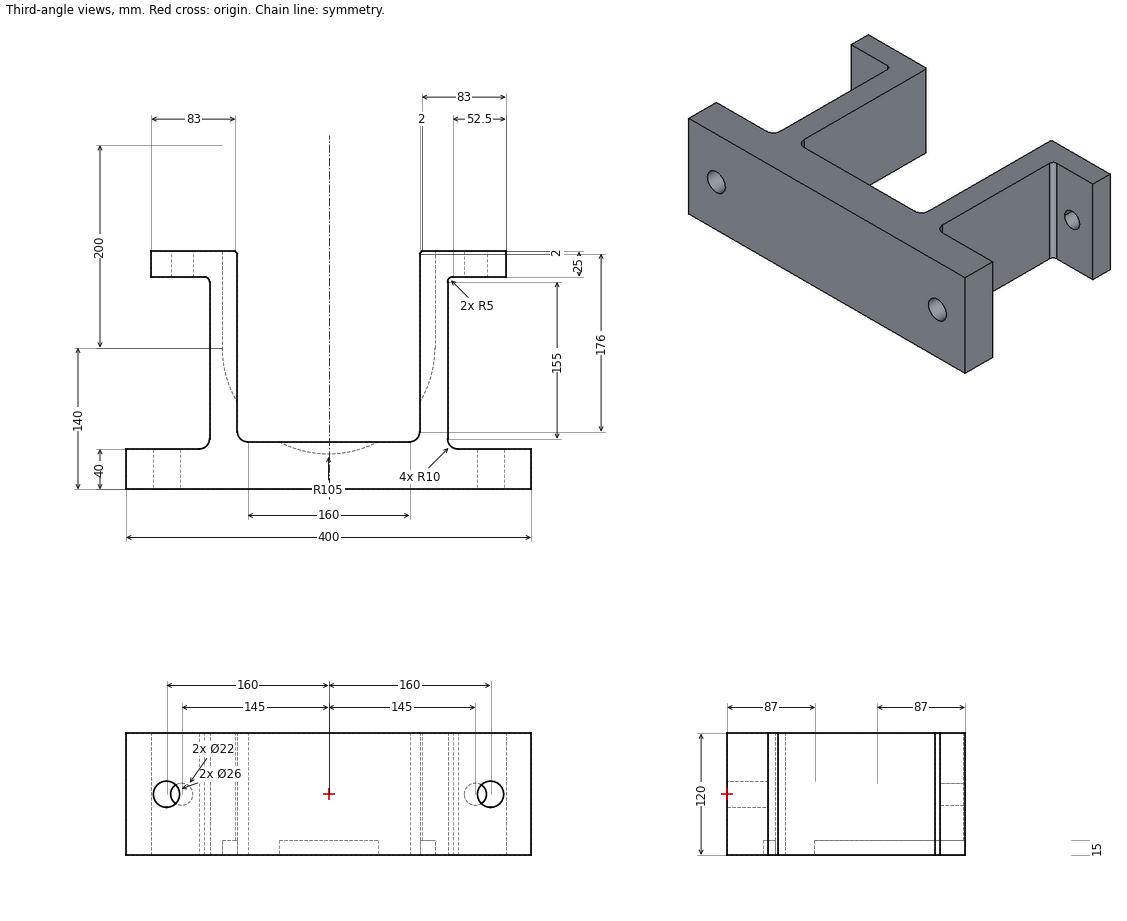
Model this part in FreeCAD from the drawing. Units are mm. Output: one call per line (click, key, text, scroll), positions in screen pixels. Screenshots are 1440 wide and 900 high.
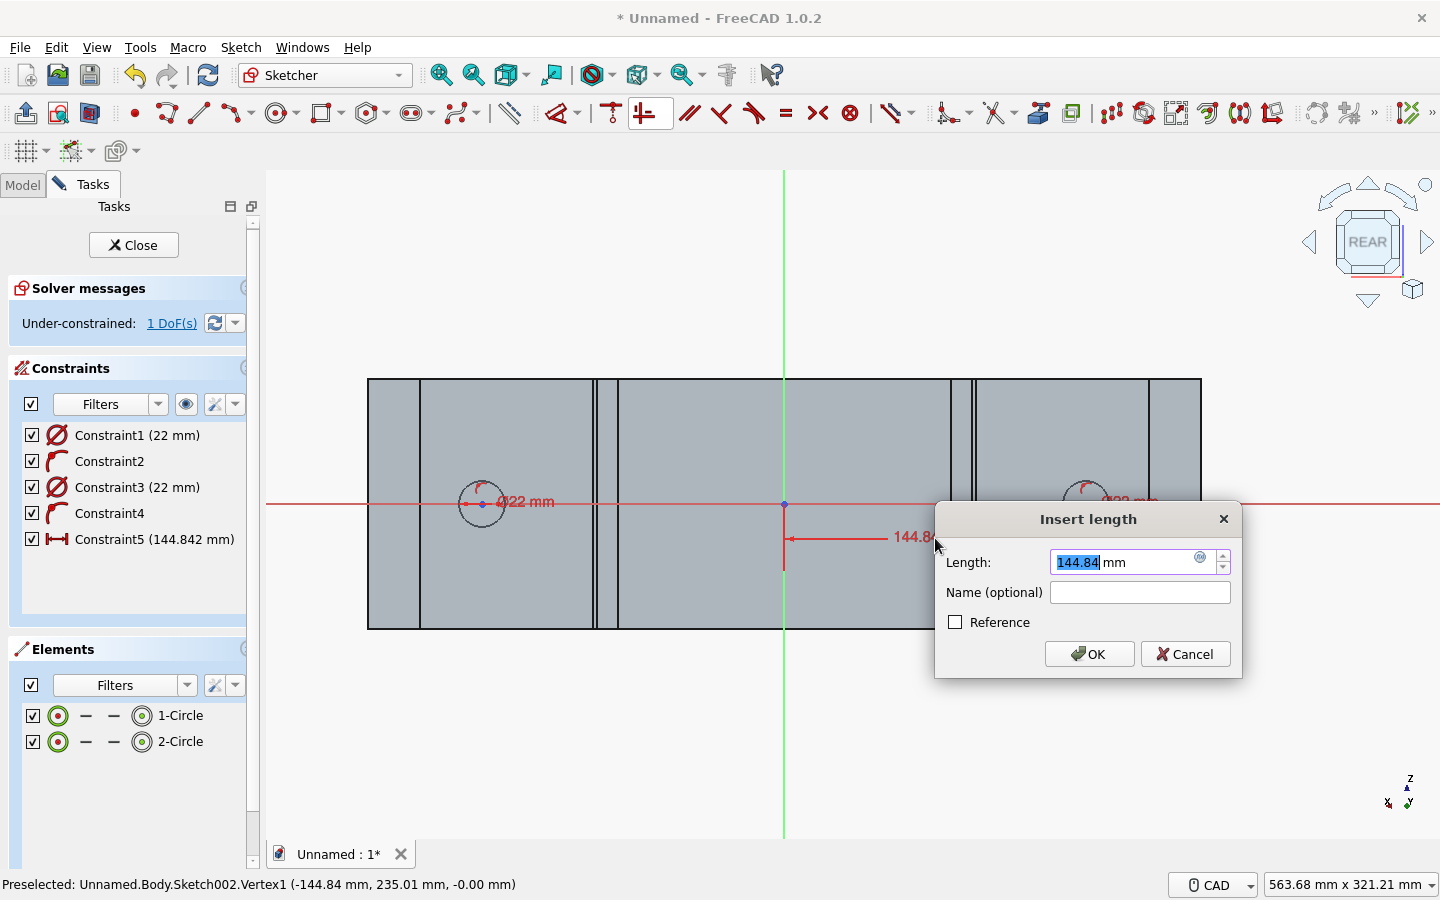
text(145)
key(Return)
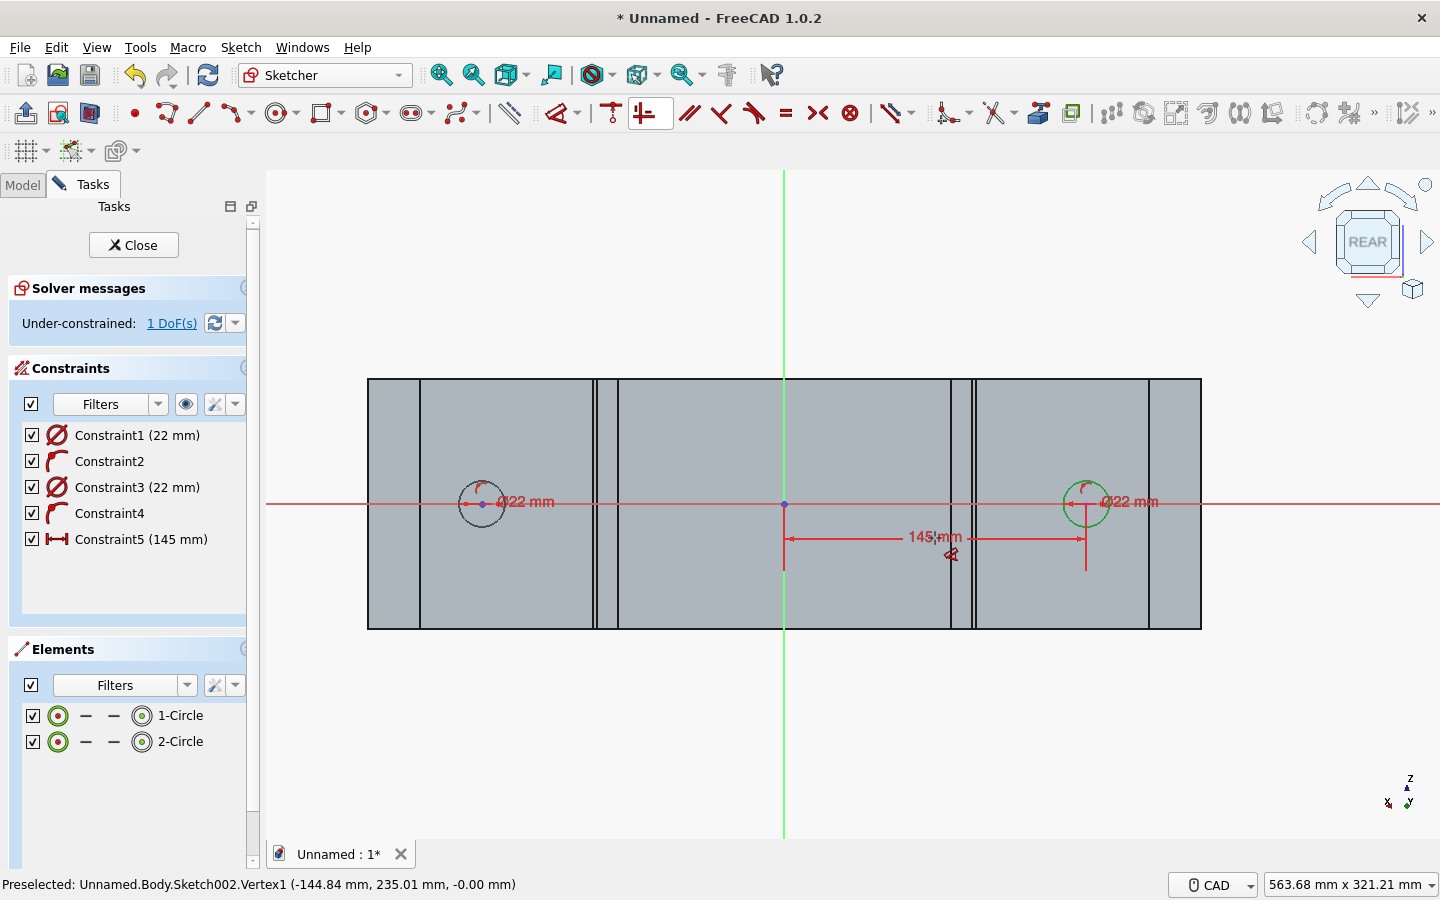
click(482, 504)
click(633, 538)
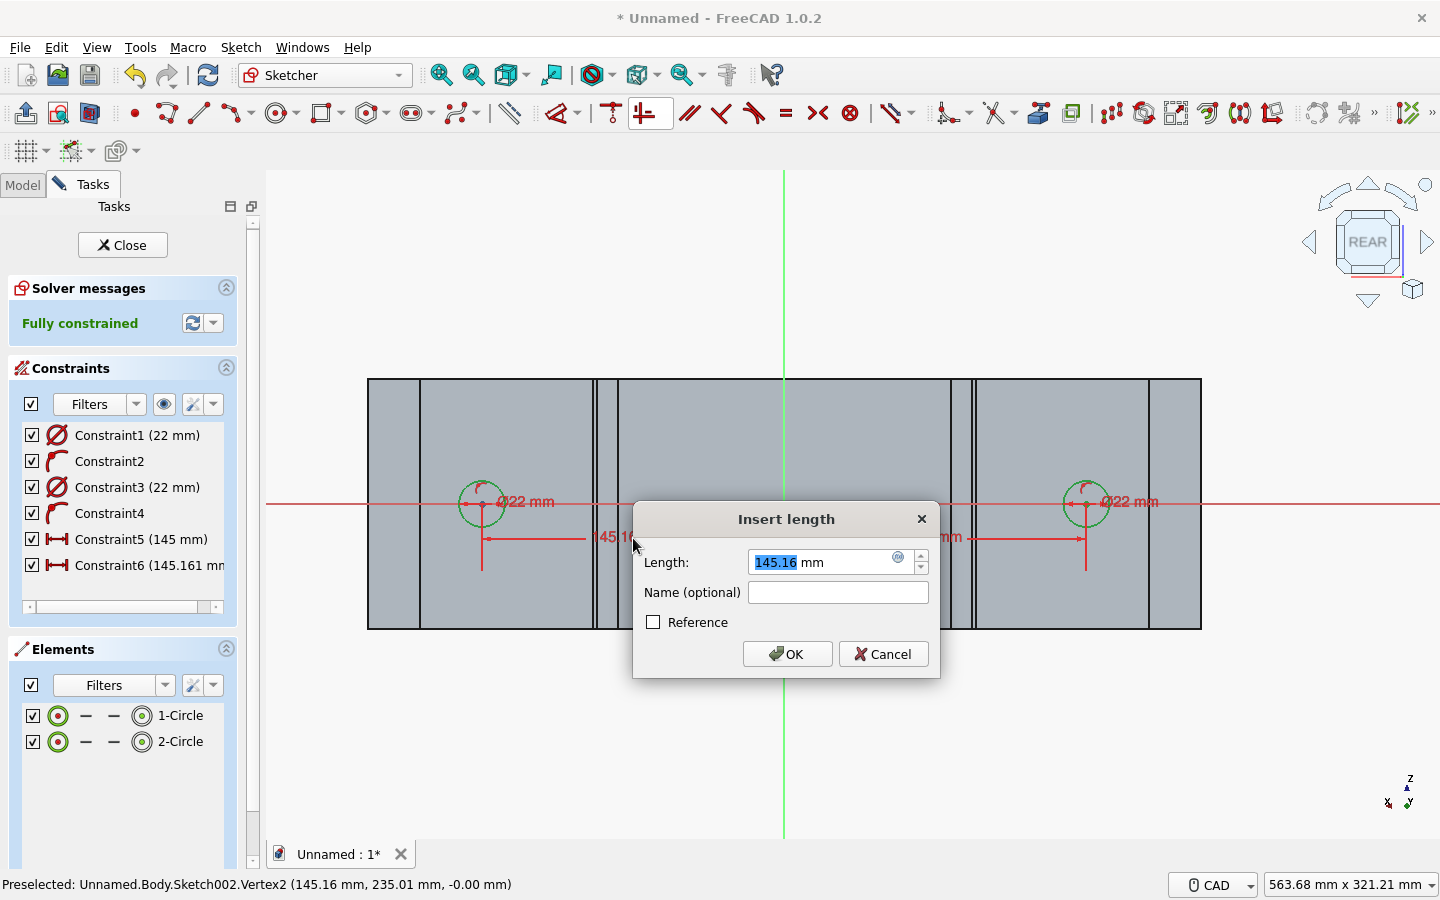
text(145)
key(Return)
key(Escape)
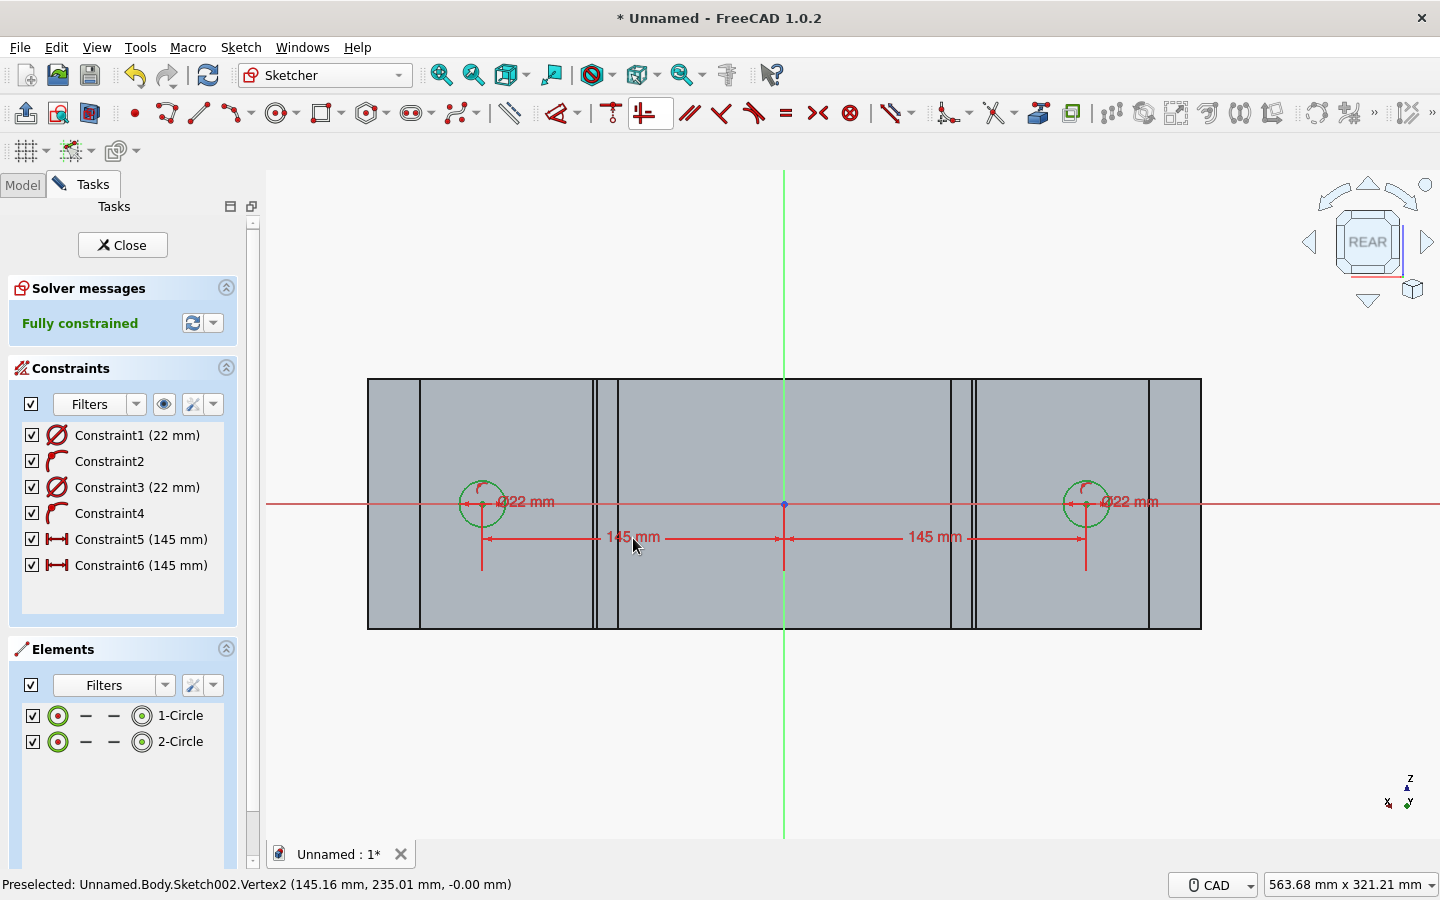
click(123, 245)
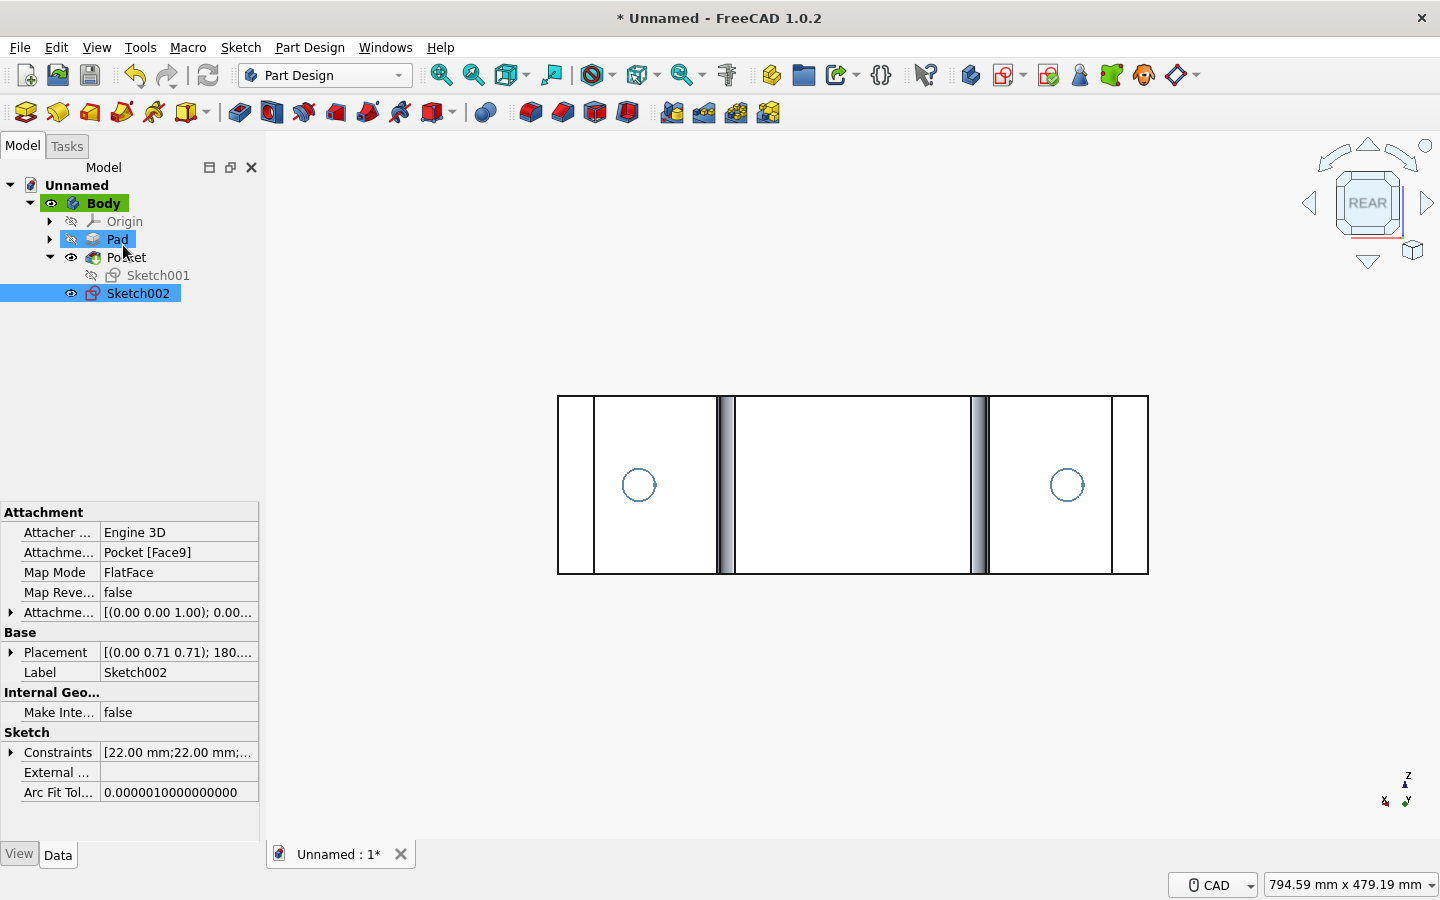
click(240, 112)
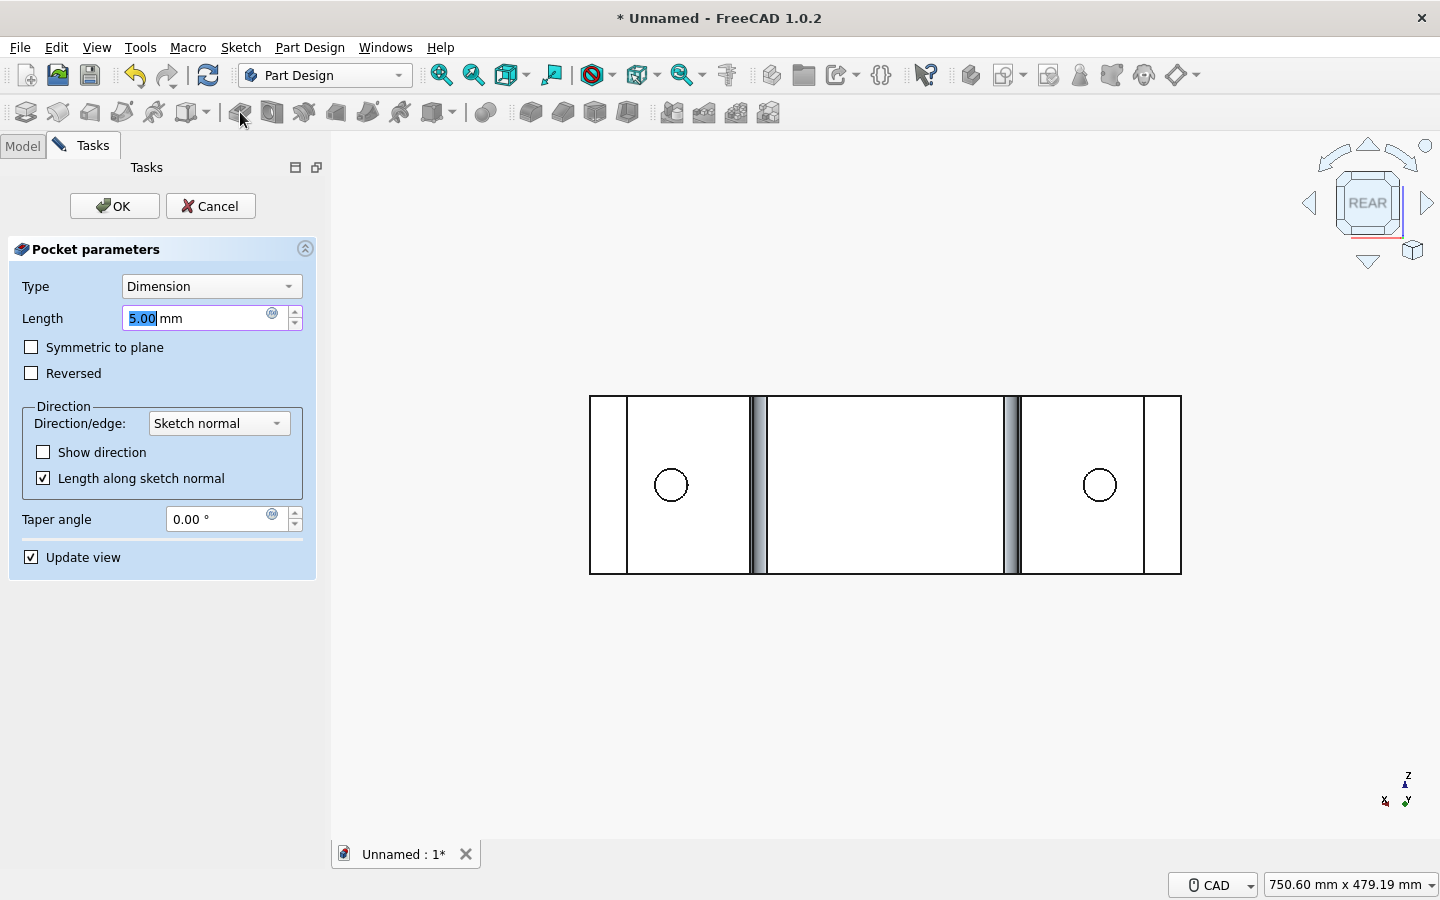
text(87)
key(Tab)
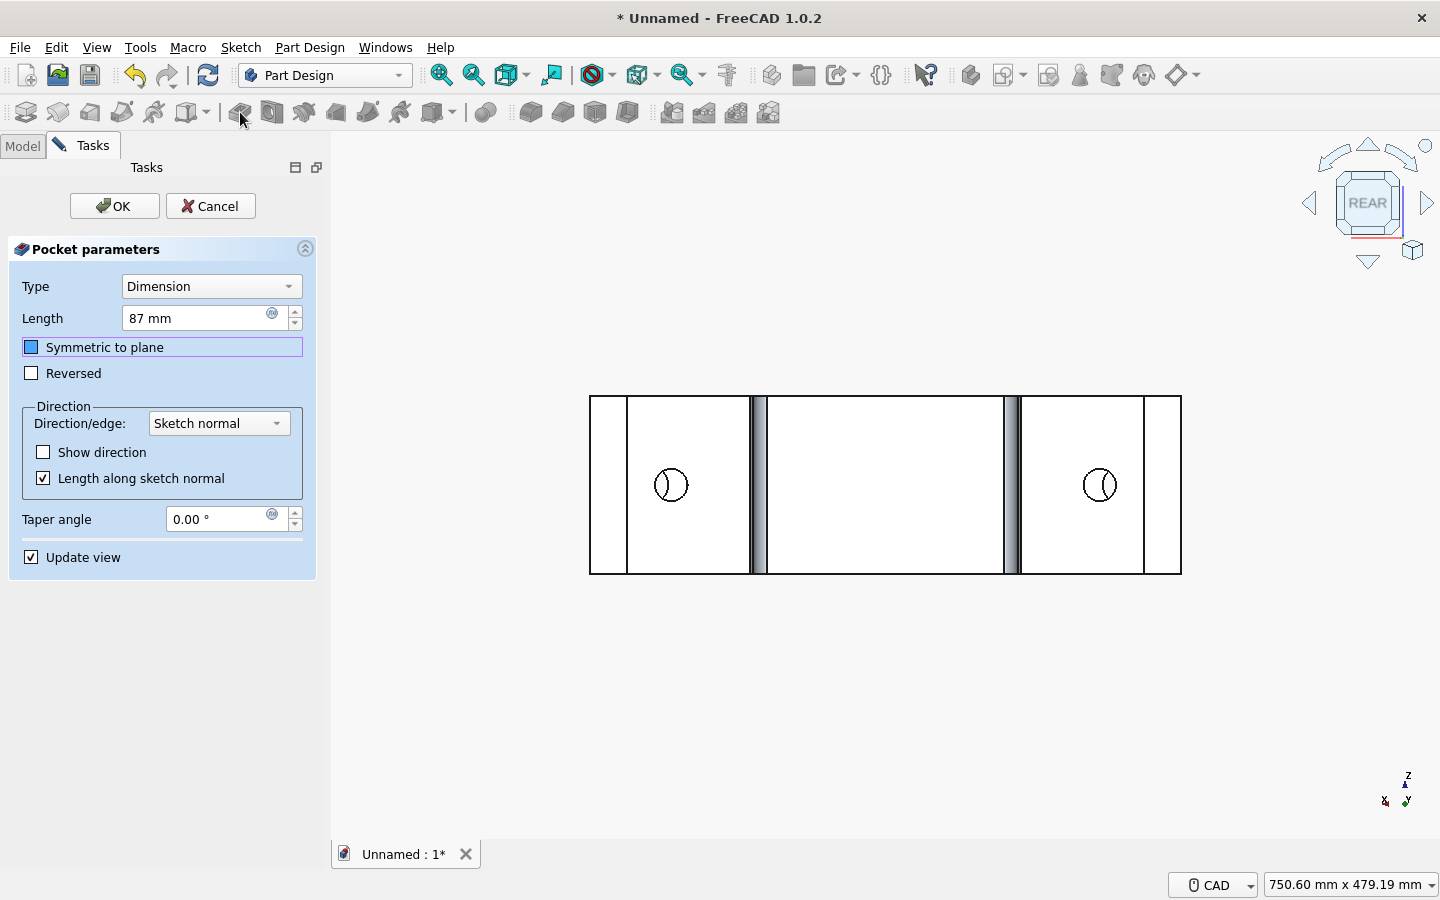
click(115, 206)